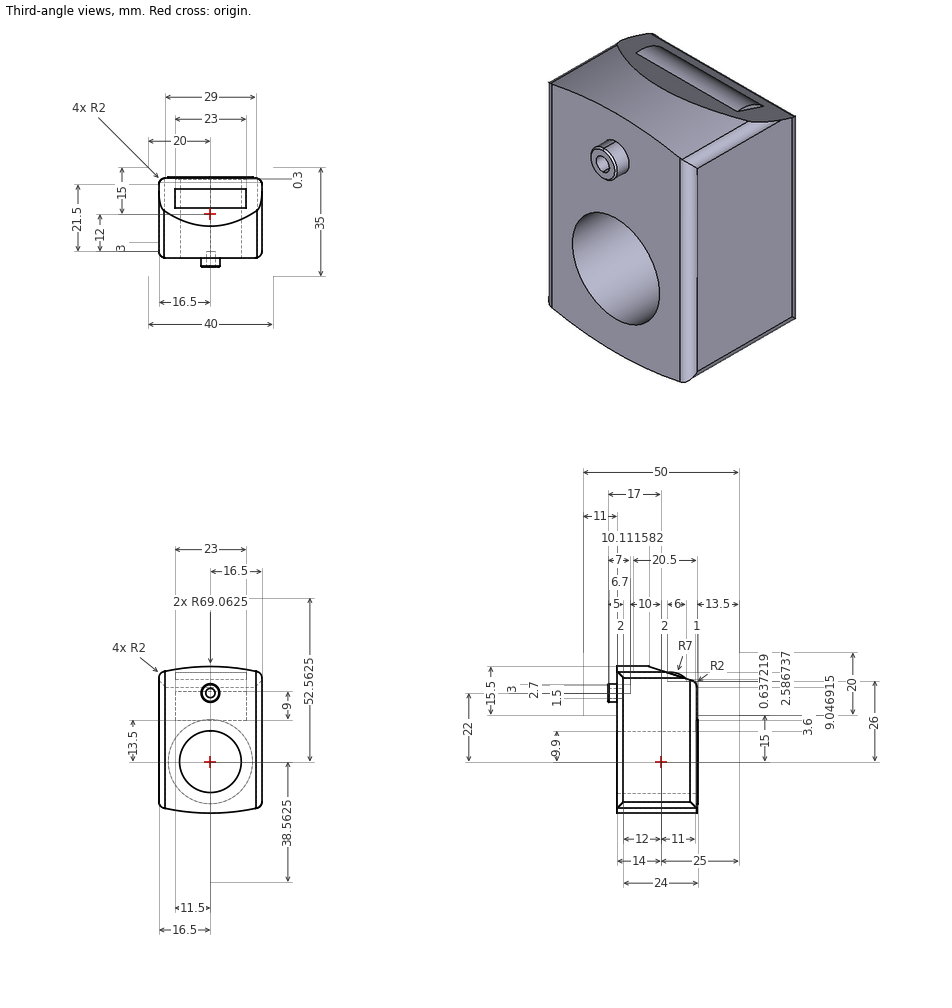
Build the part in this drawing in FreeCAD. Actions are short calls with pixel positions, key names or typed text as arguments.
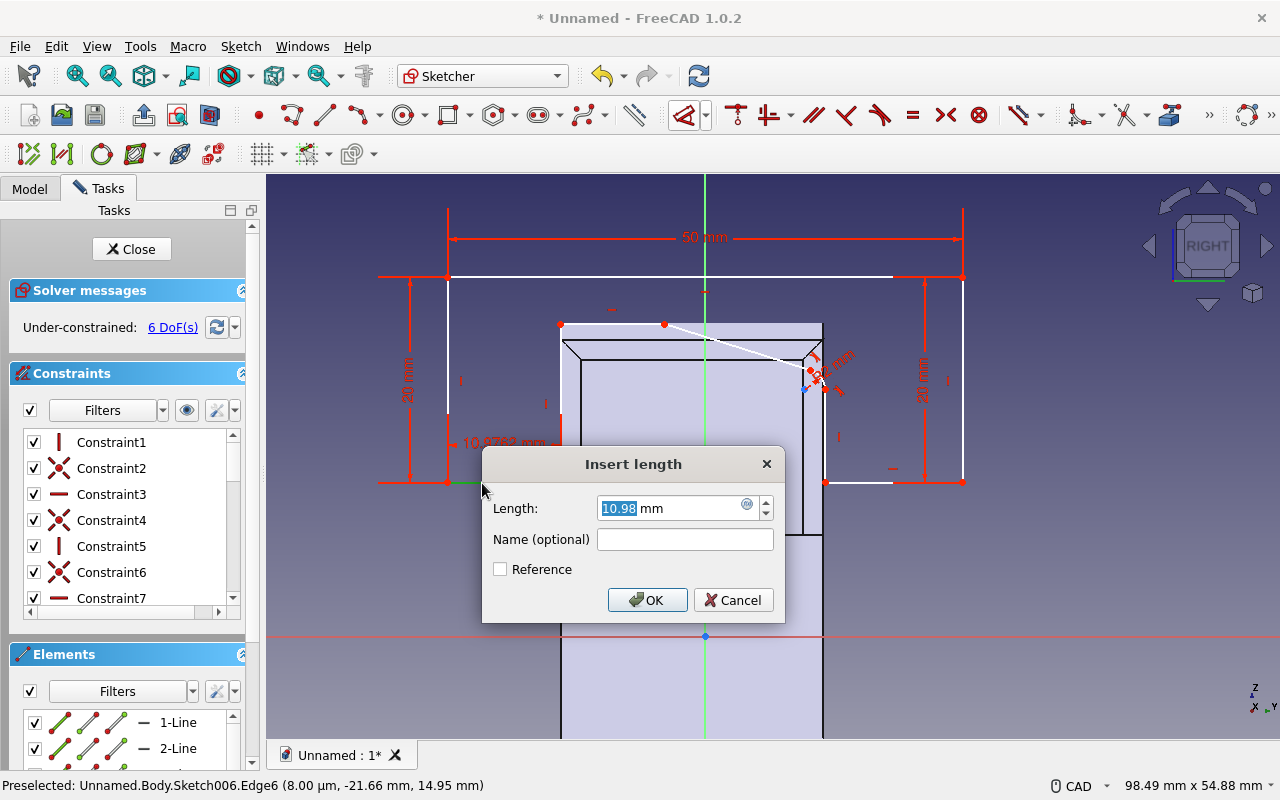
text(11)
key(Return)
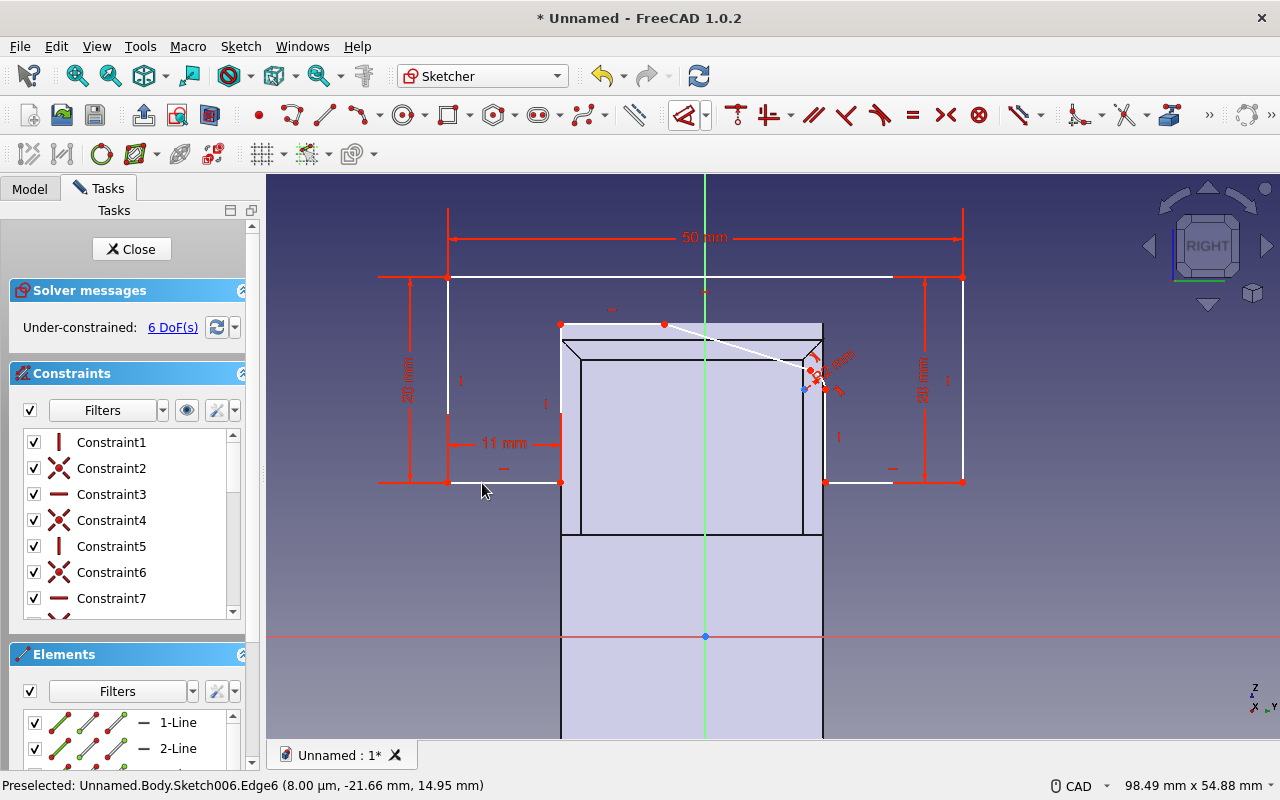
click(825, 483)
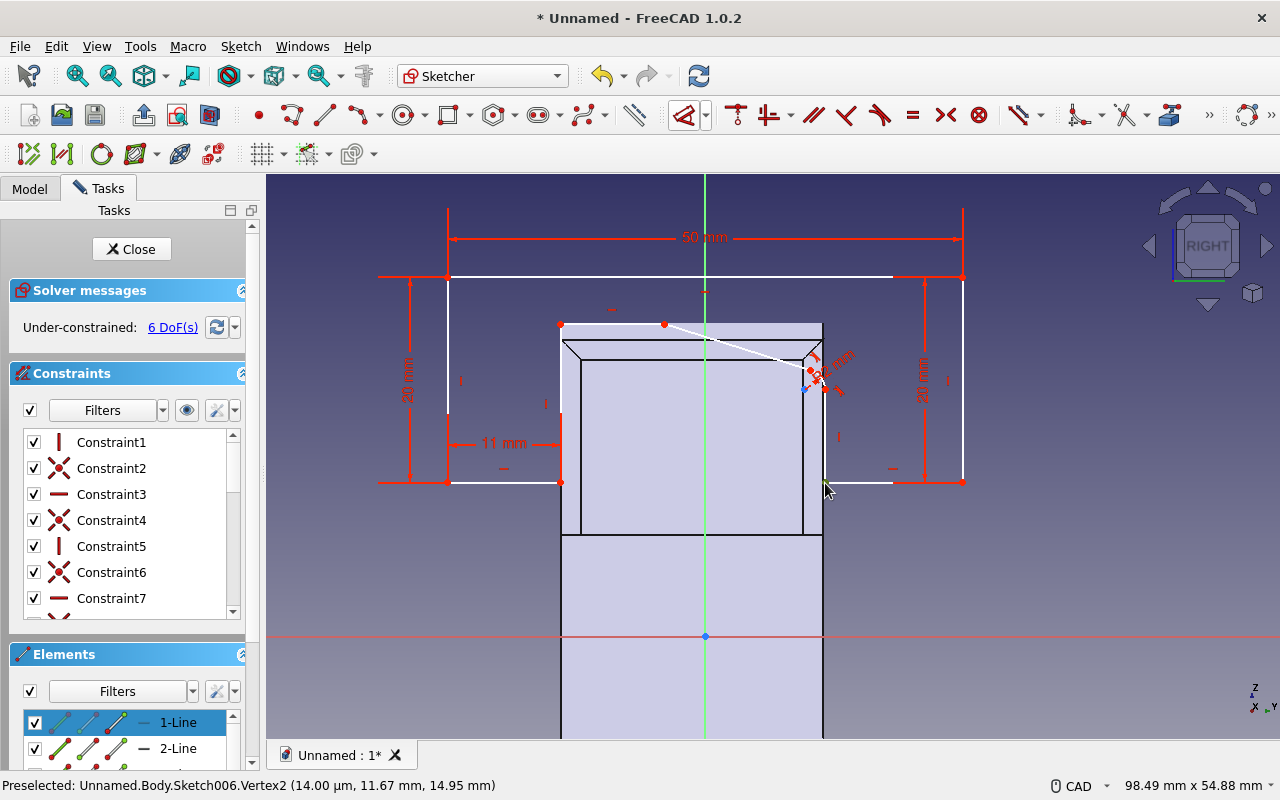
click(706, 116)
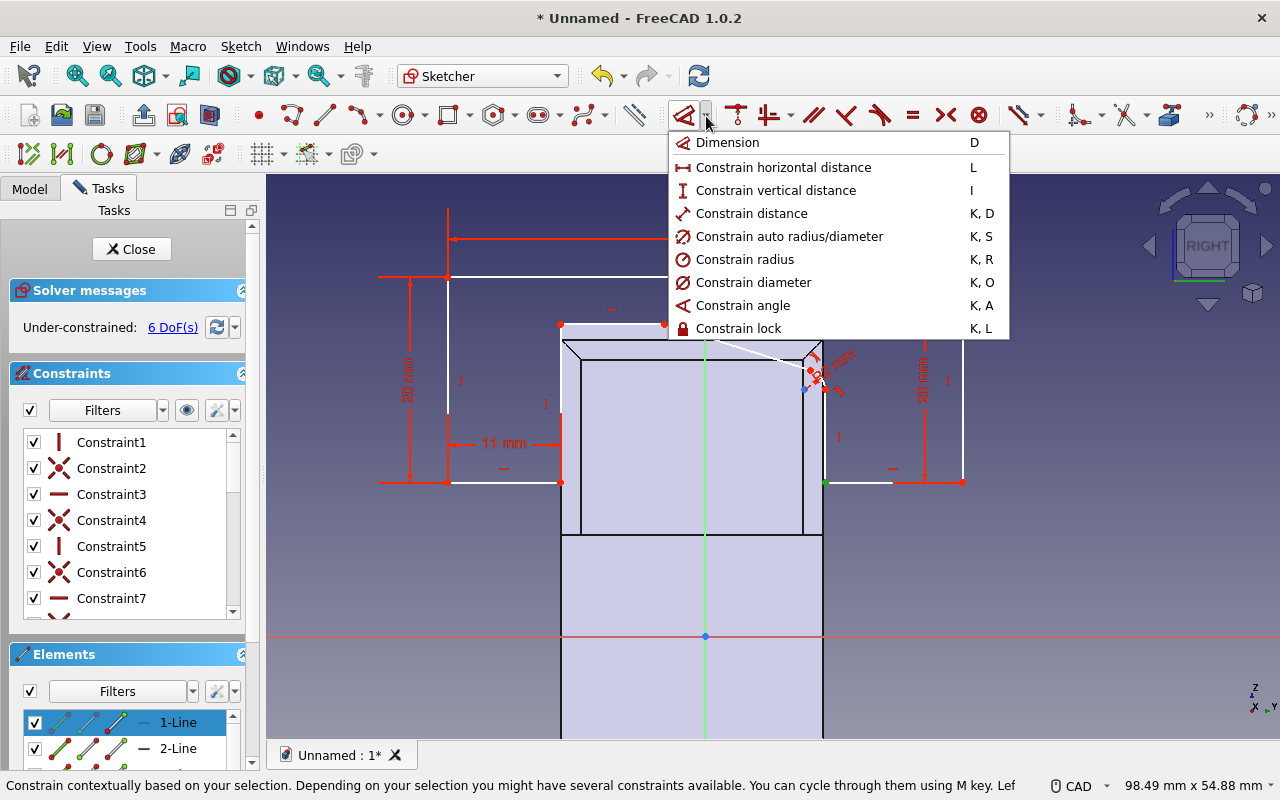
click(839, 190)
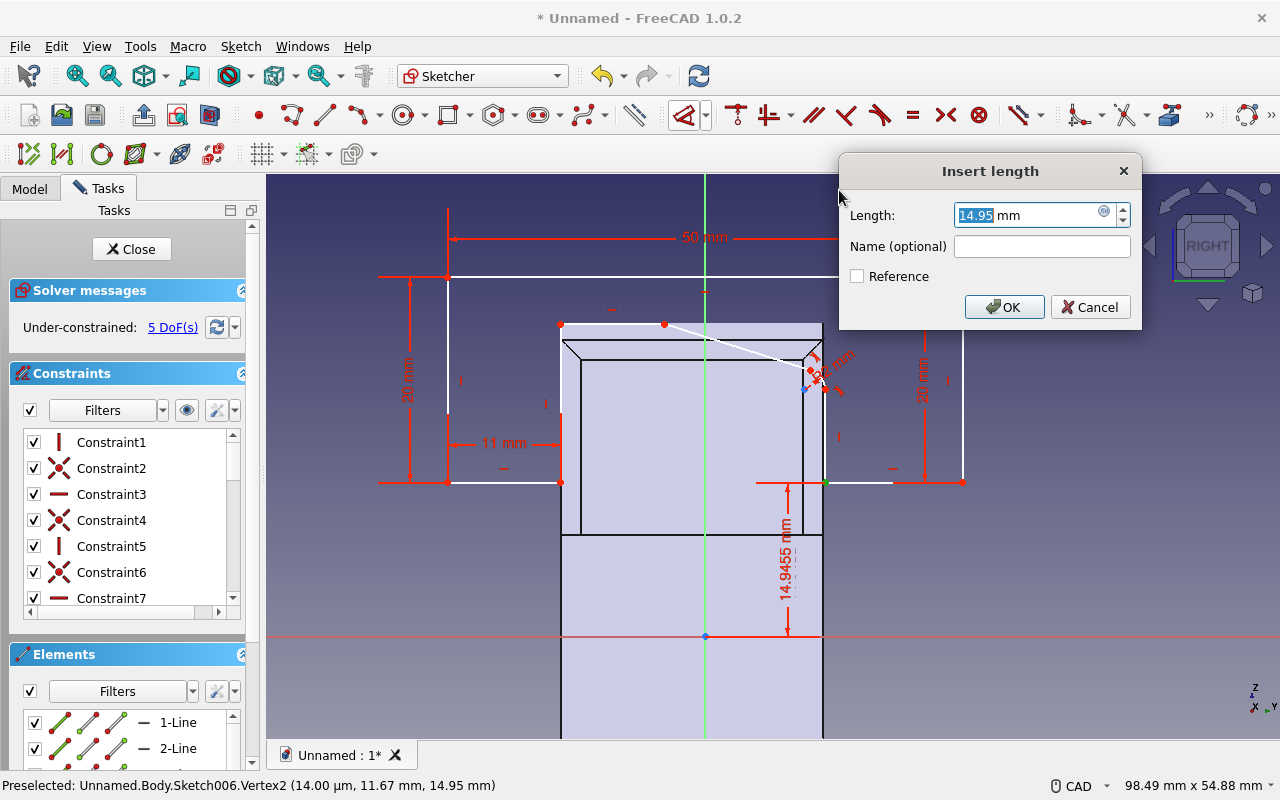
text(15)
key(Return)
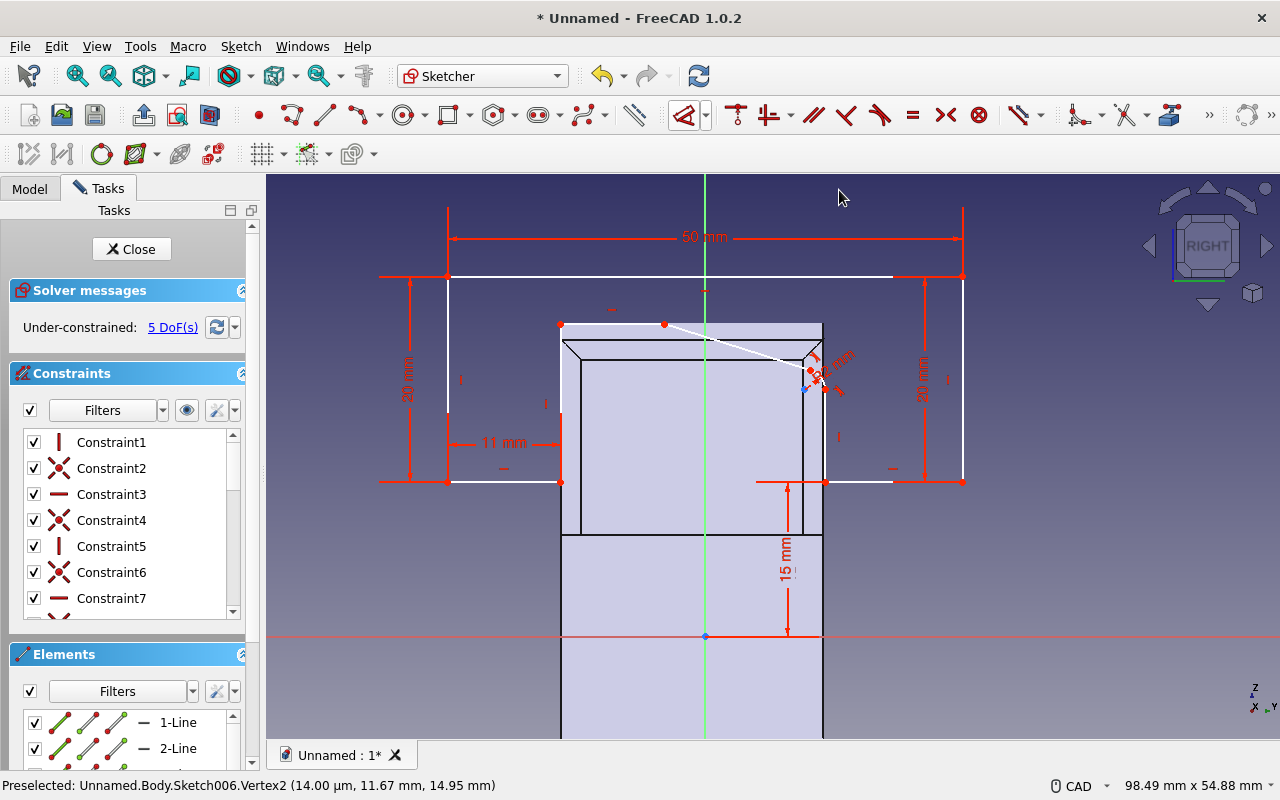
click(963, 482)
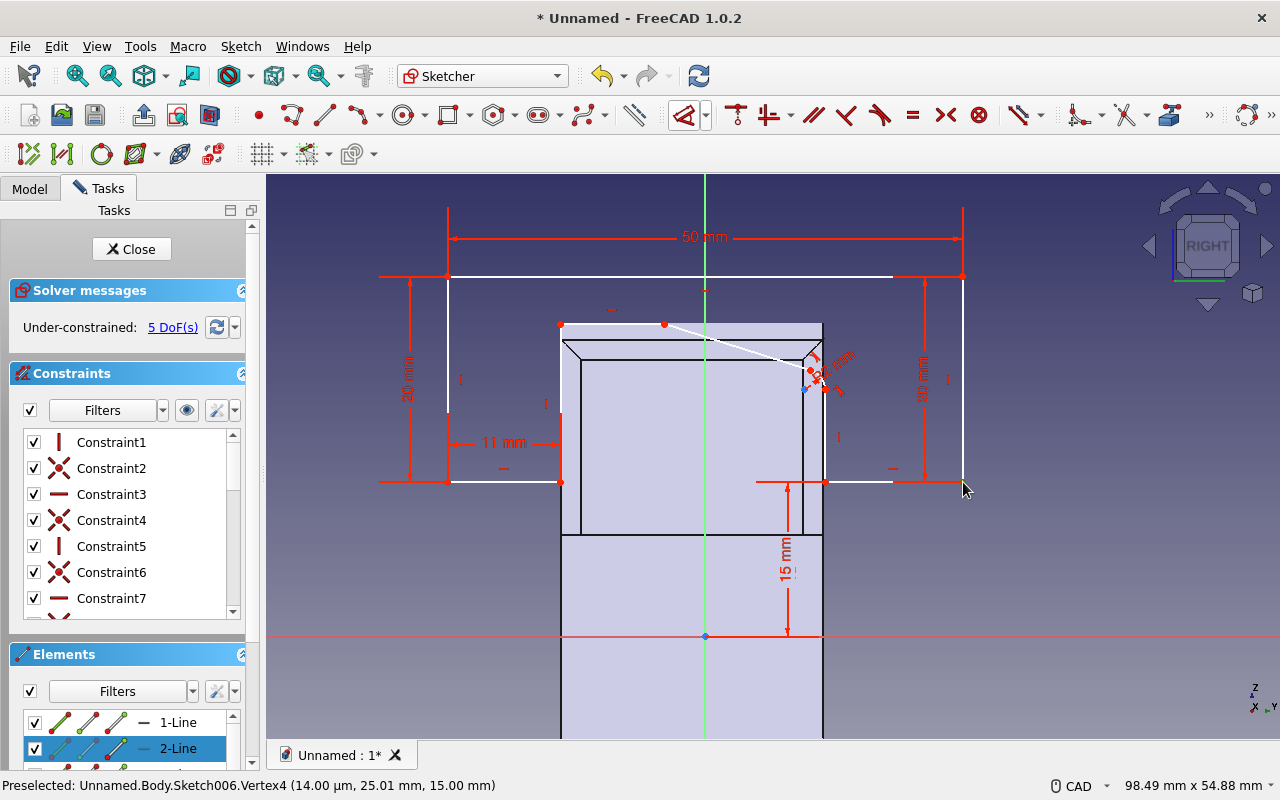
click(706, 116)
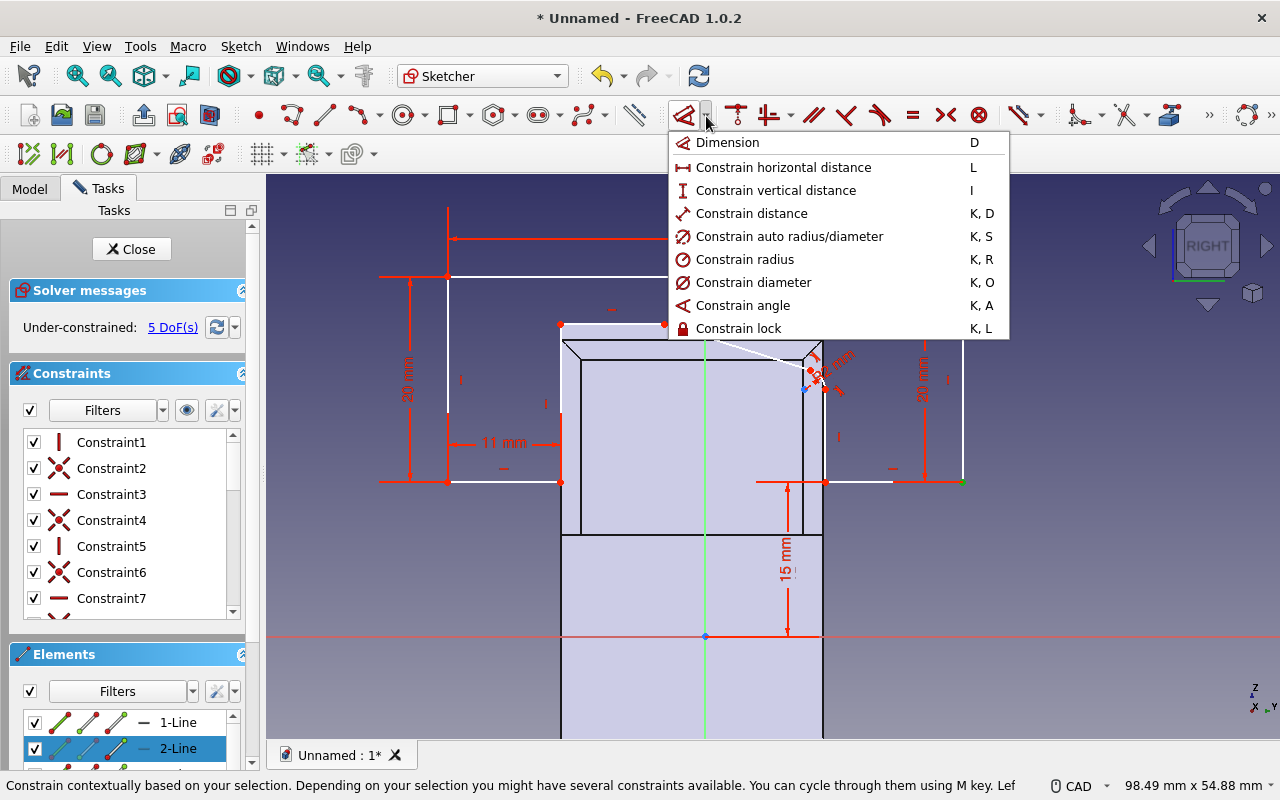
click(839, 168)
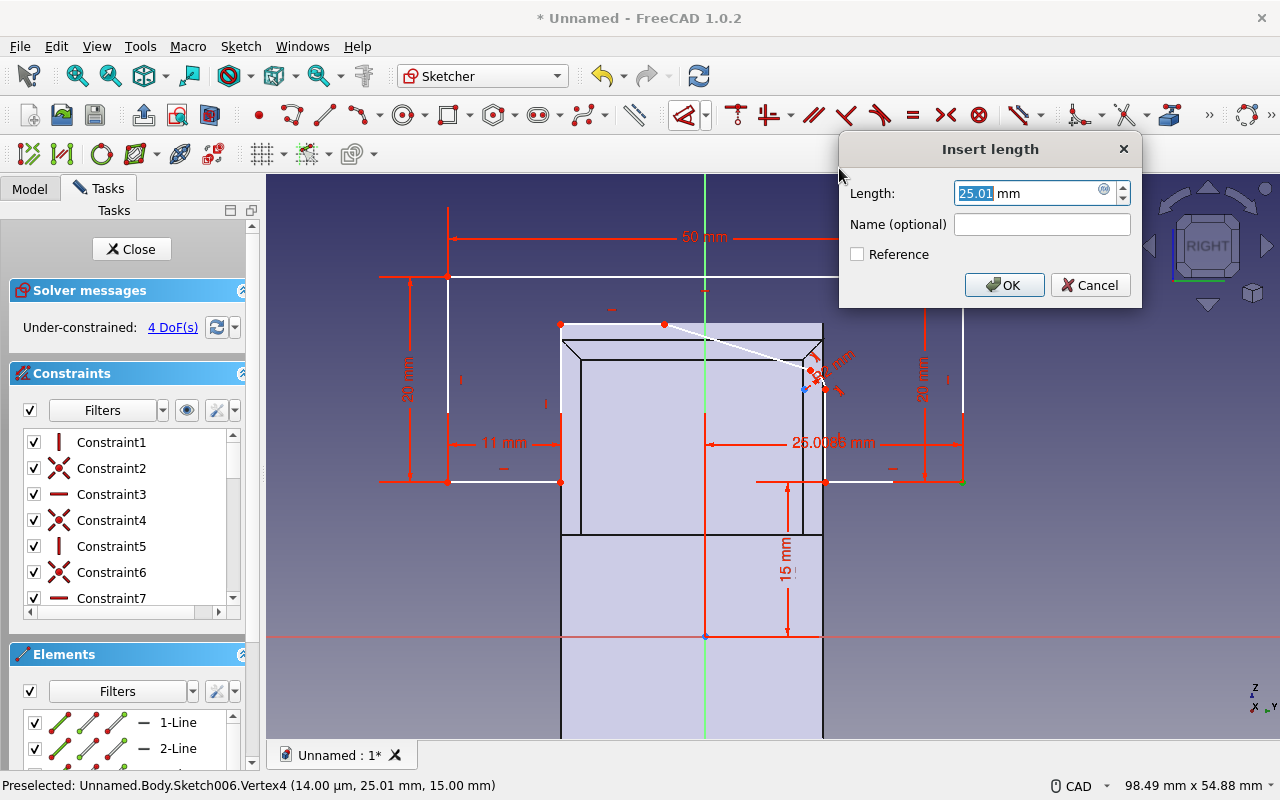
text(25)
key(Return)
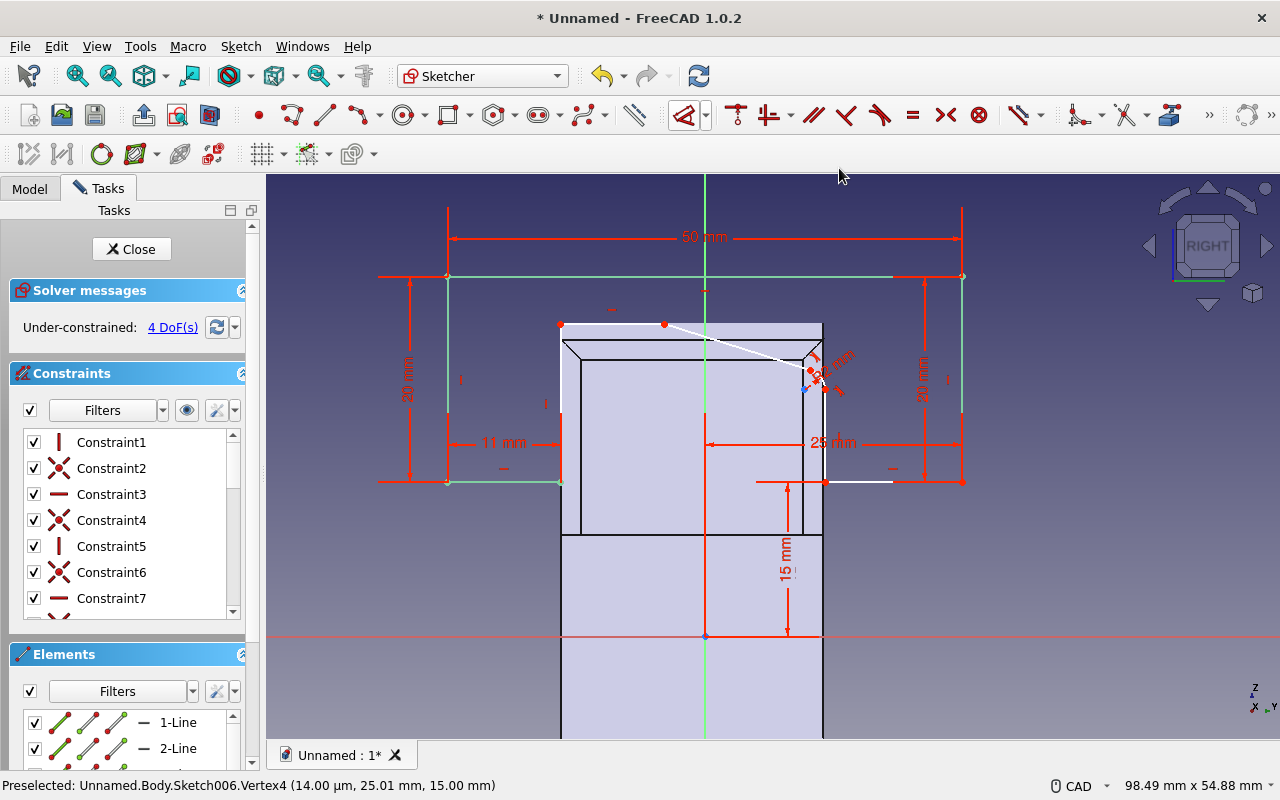
click(866, 482)